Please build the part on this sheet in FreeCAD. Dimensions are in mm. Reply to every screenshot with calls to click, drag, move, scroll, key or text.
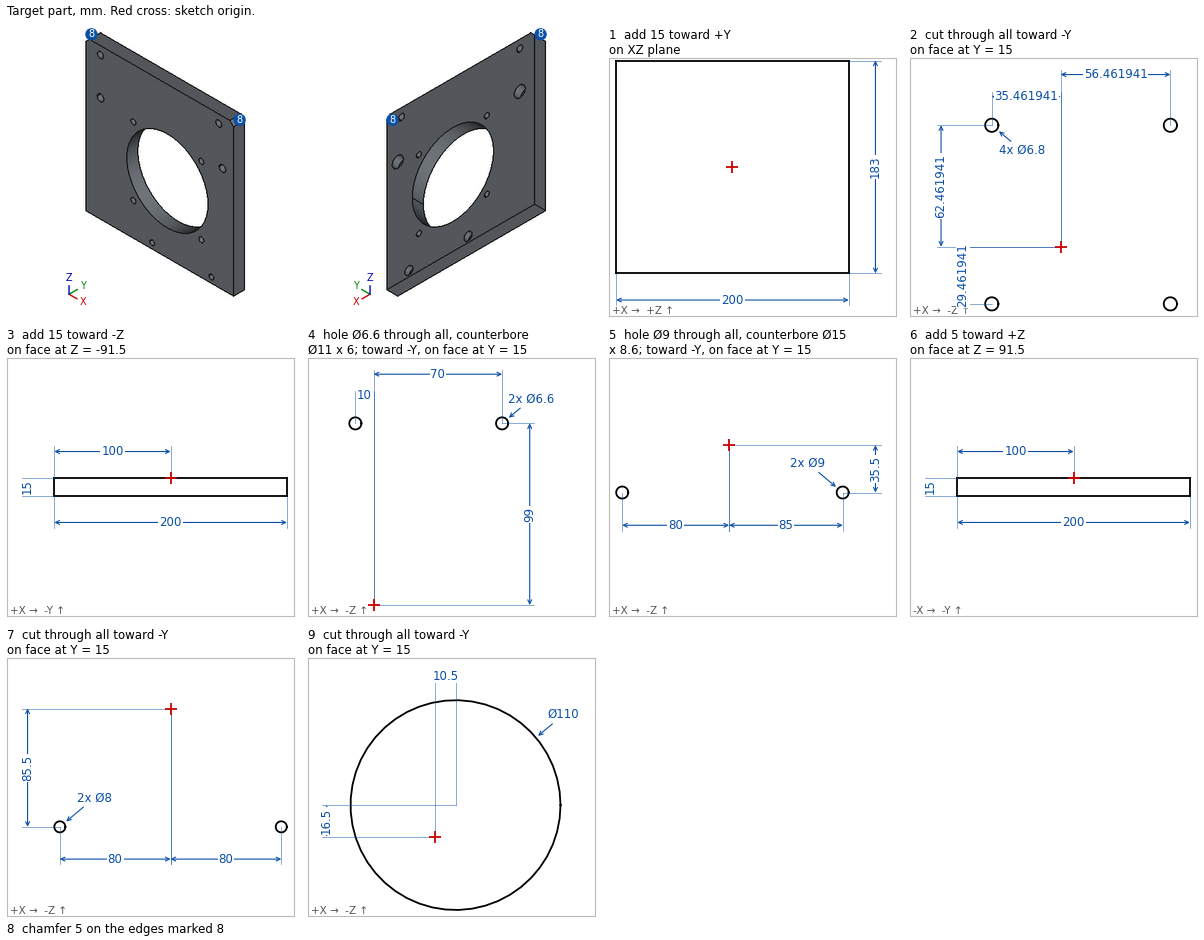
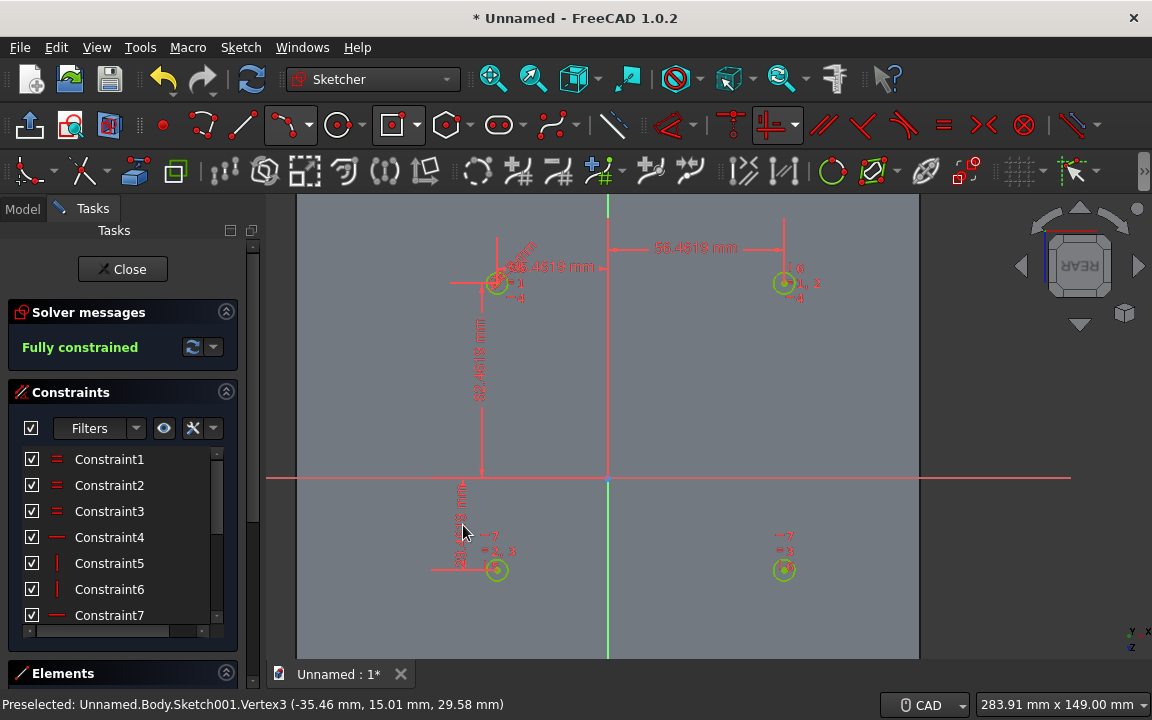
click(123, 269)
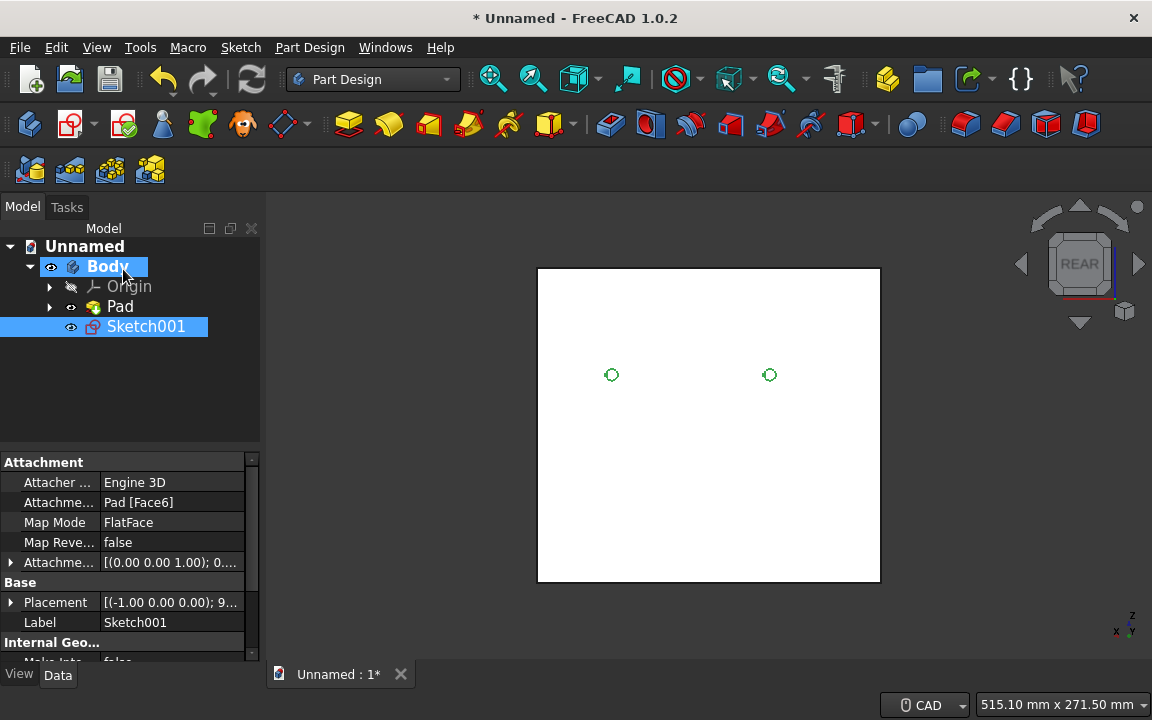
click(612, 124)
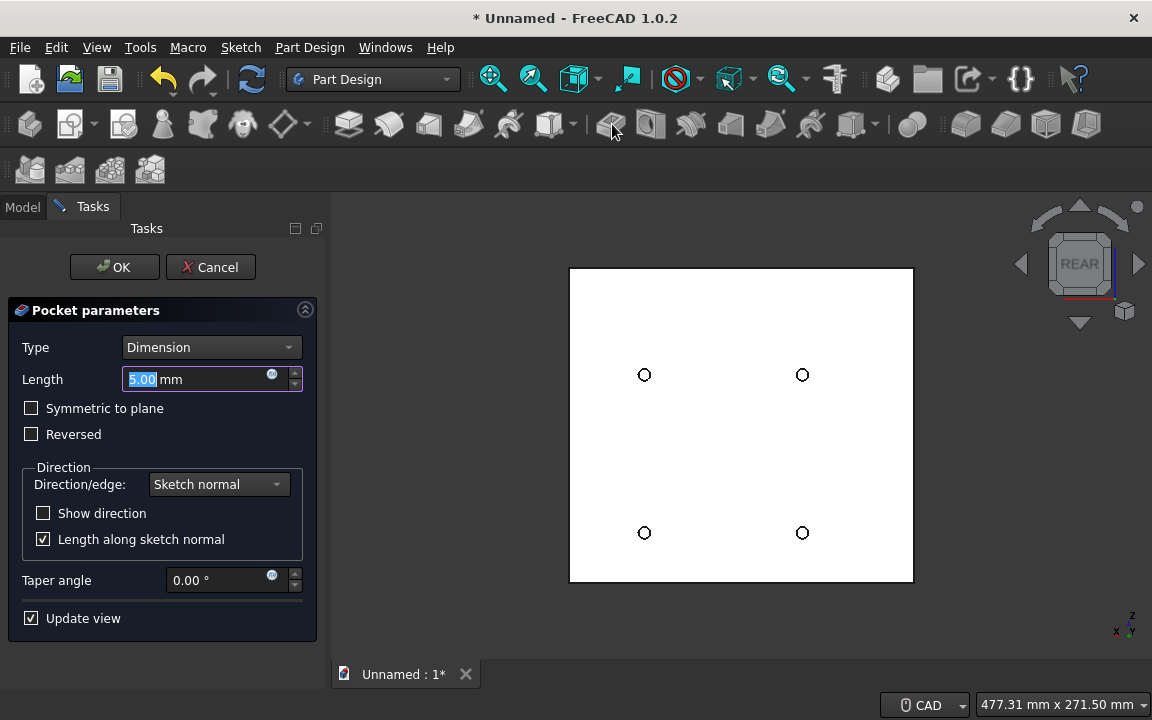
click(212, 348)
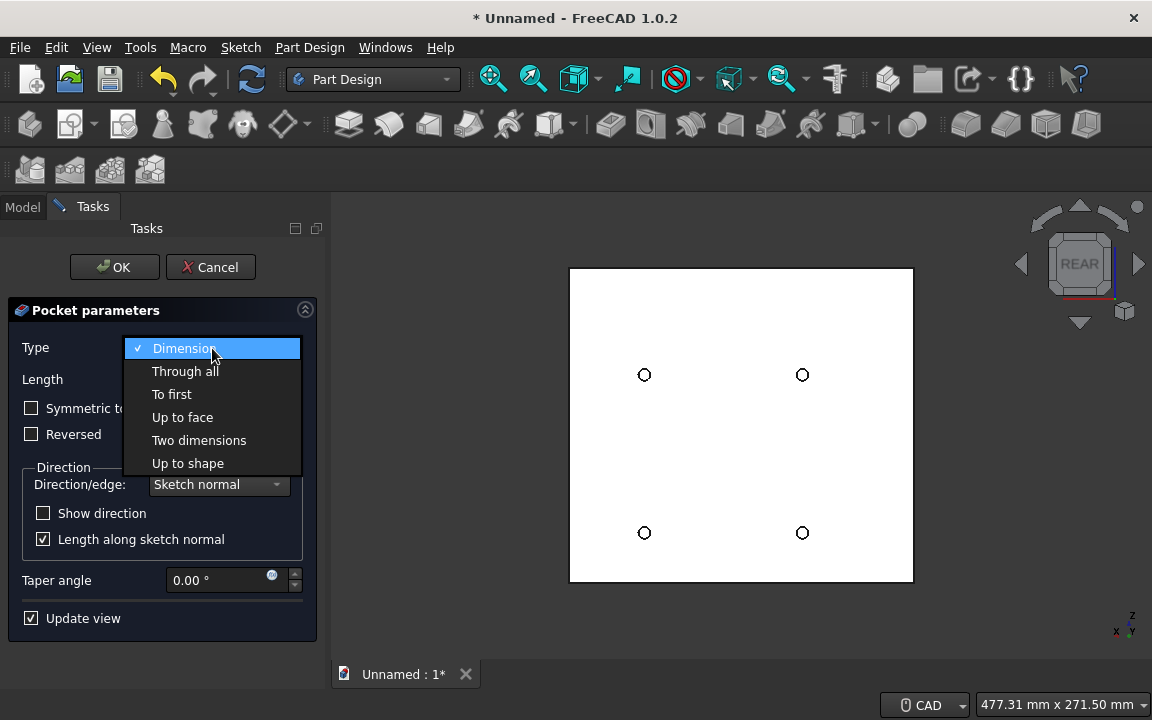
click(212, 372)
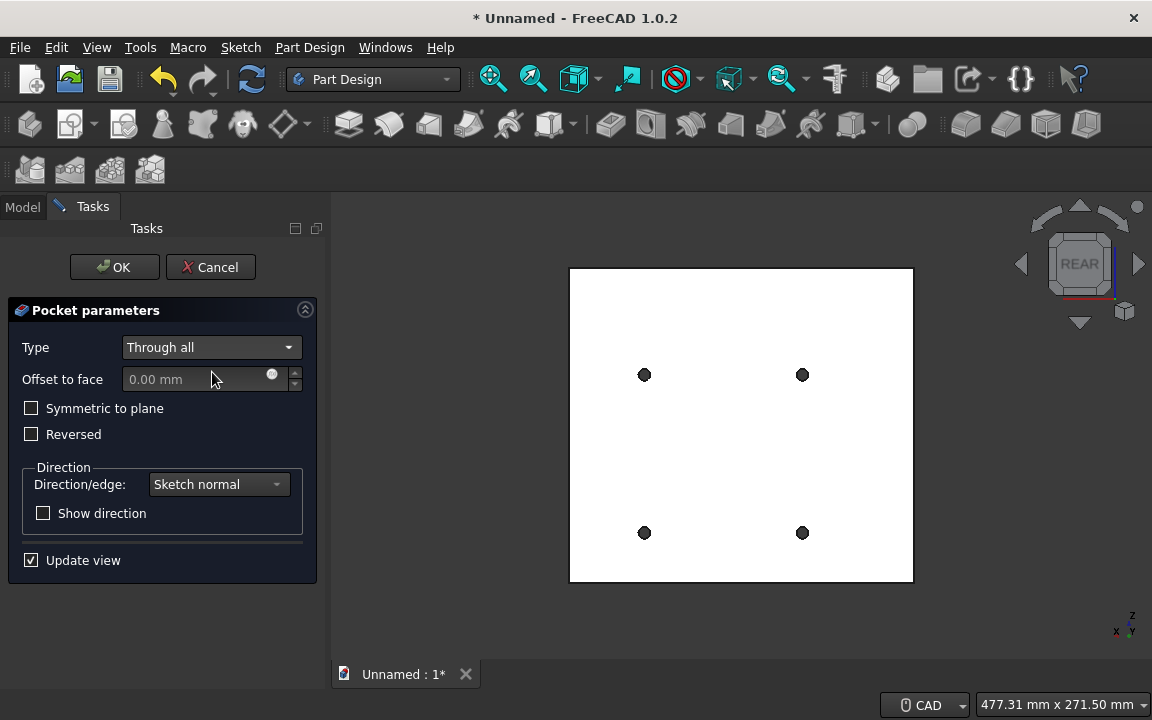
click(115, 267)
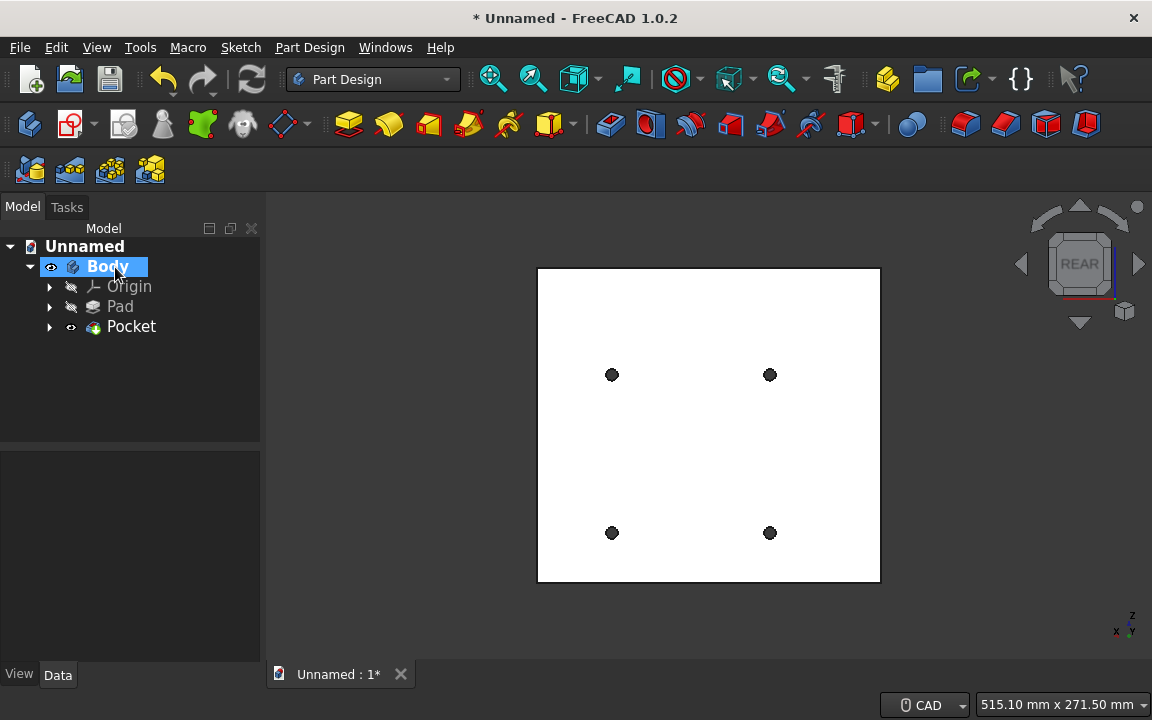
key(5)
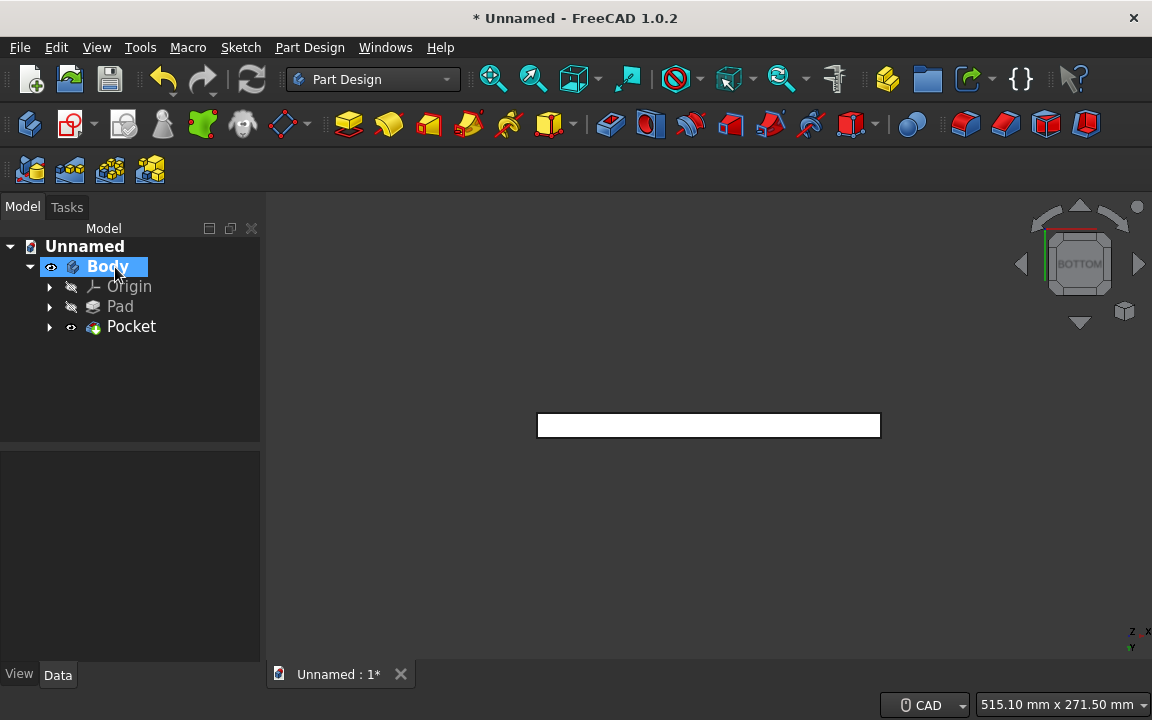
click(494, 80)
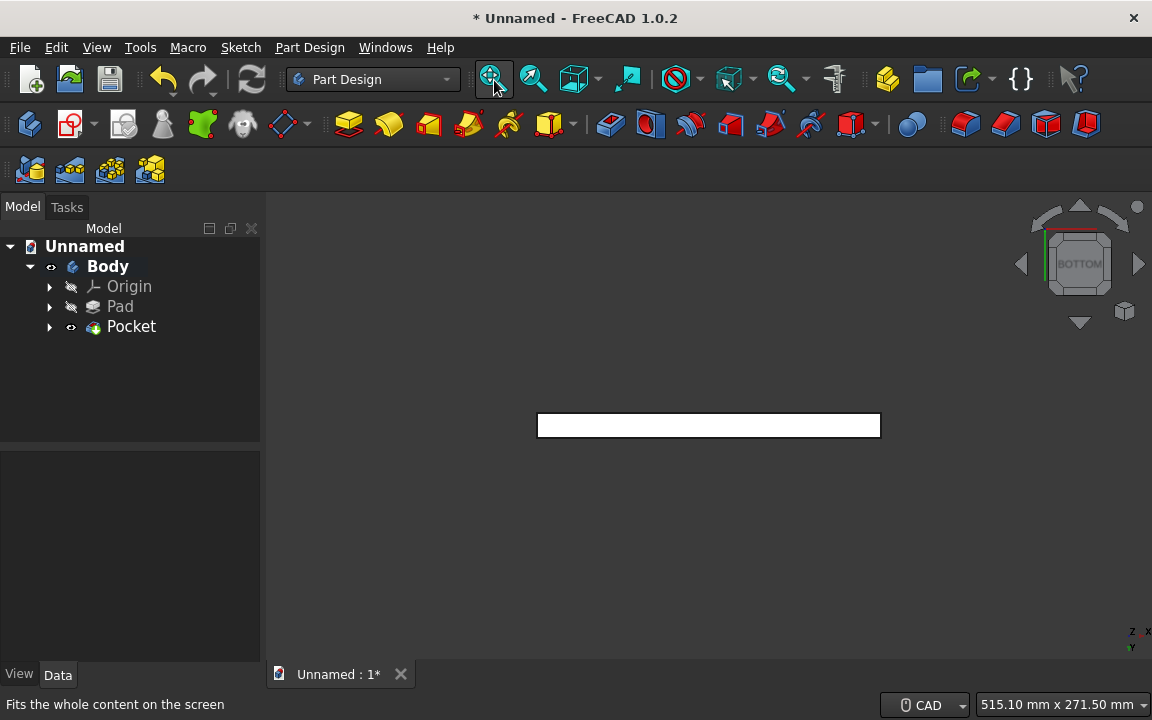
click(856, 424)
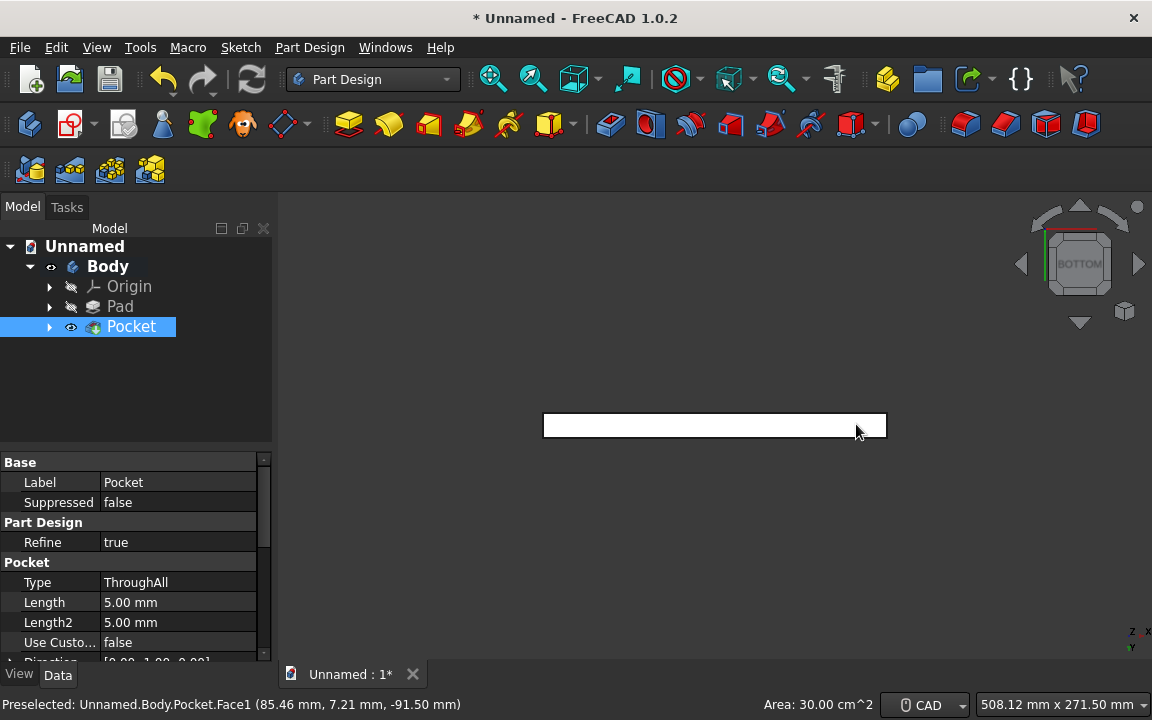
click(70, 124)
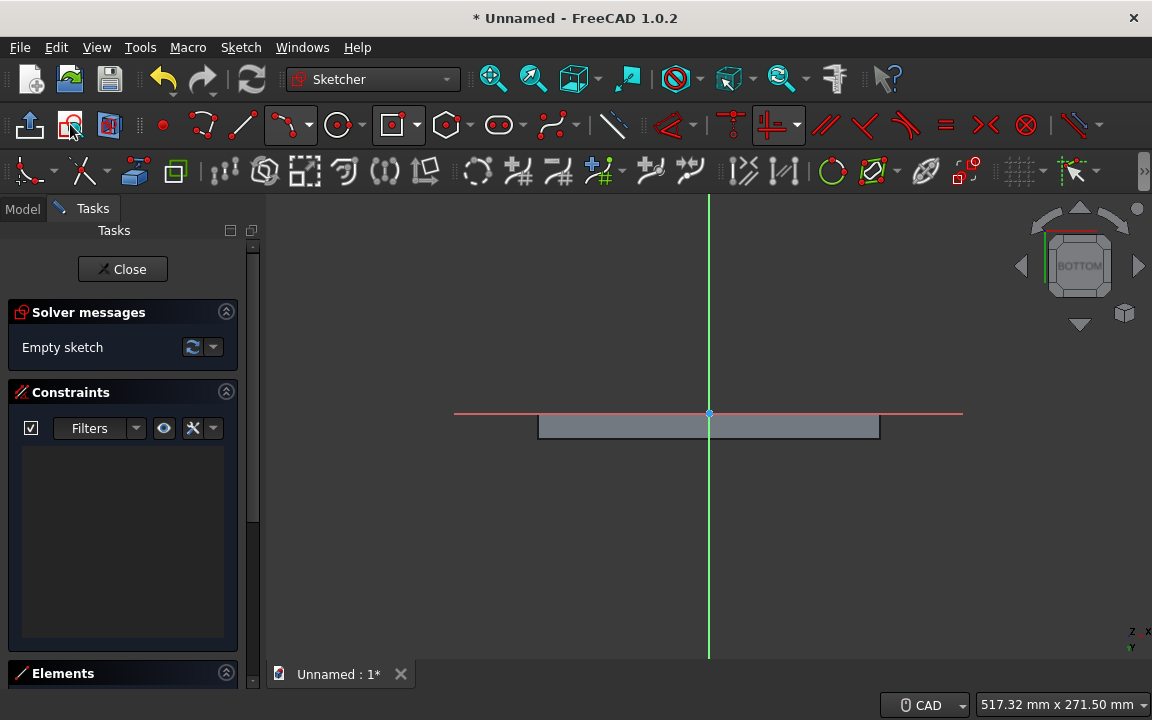
scroll(848, 426, up, 2)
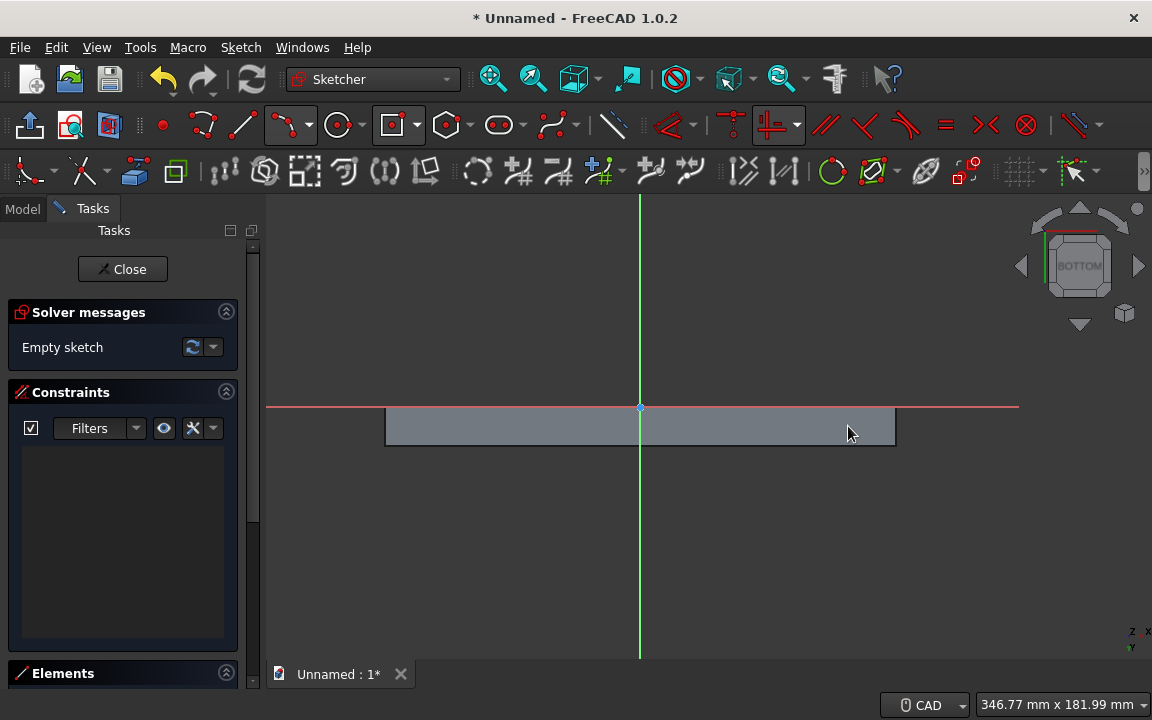
key(g)
key(r)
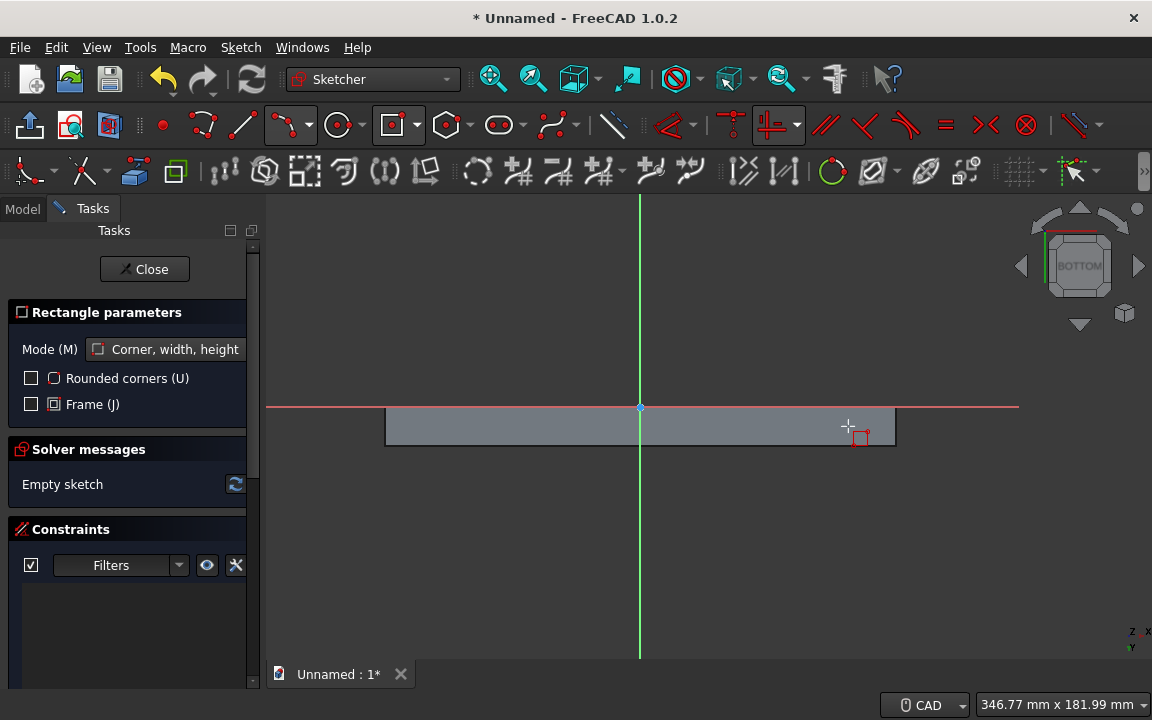
click(385, 407)
click(896, 446)
key(Escape)